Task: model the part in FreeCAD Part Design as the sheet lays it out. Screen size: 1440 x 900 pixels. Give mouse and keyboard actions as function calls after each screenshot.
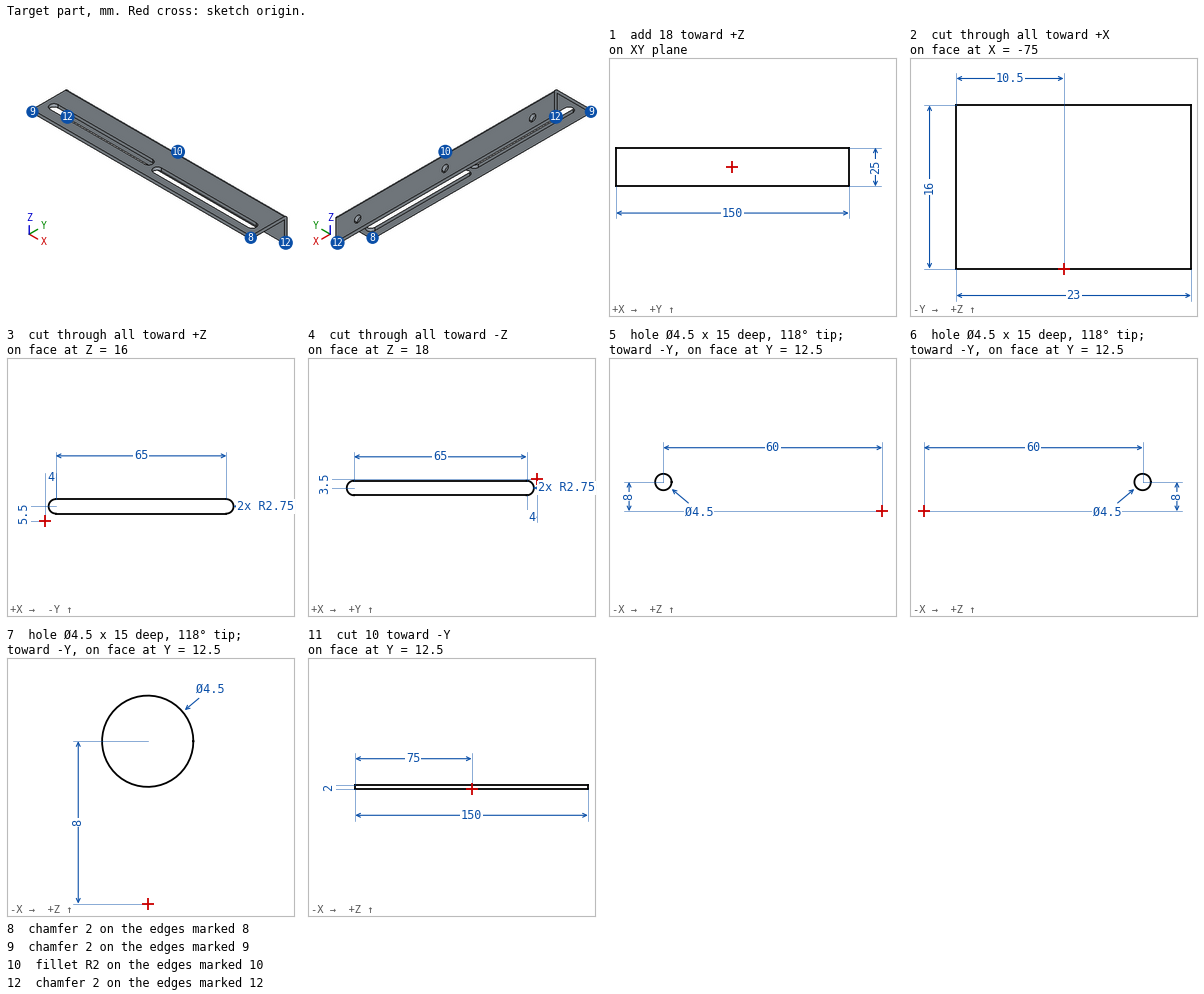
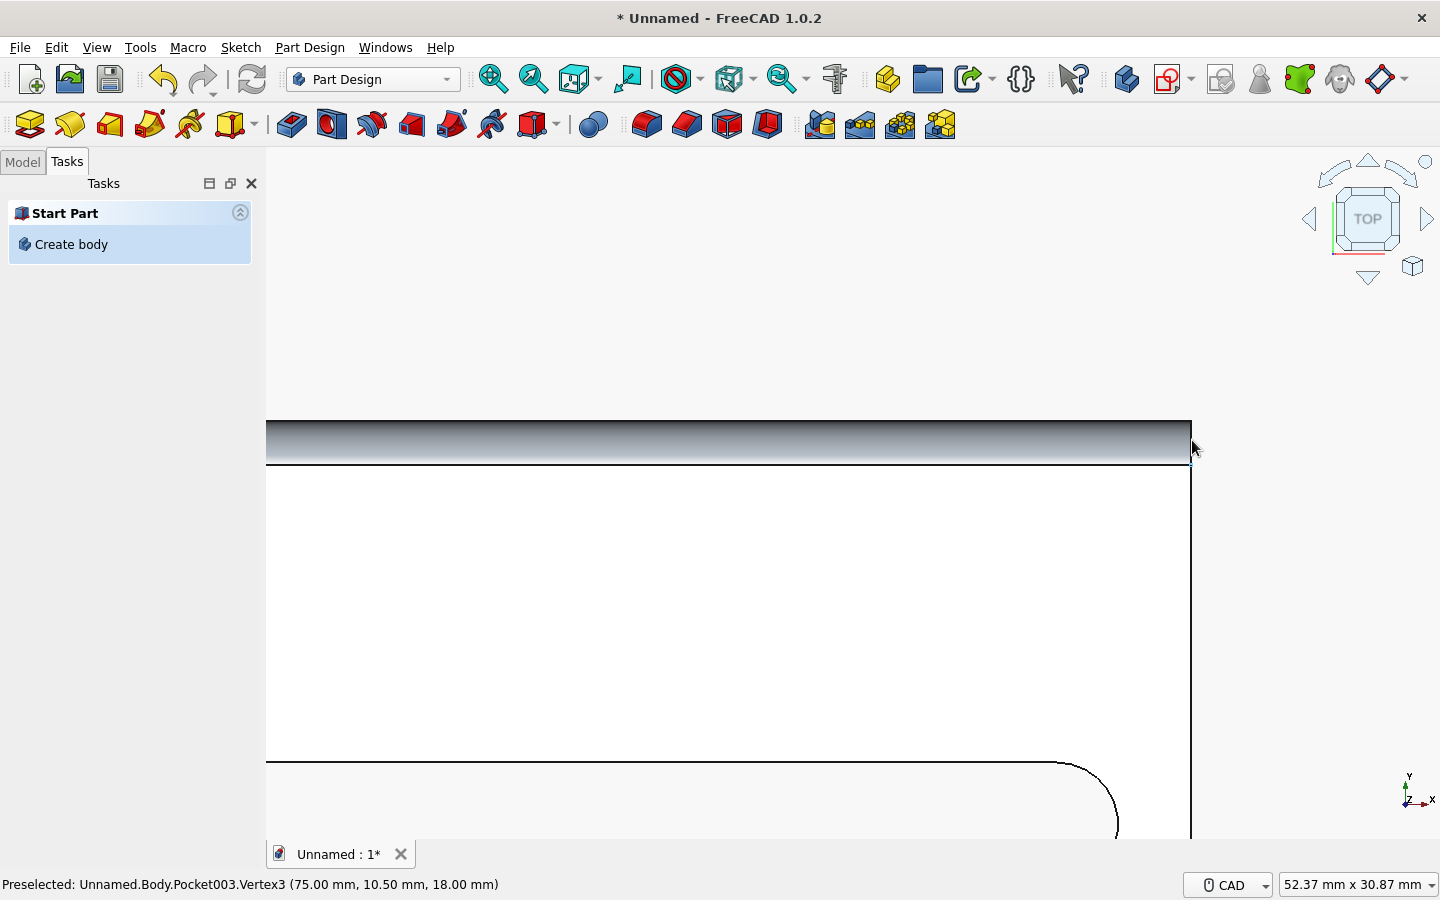
click(494, 80)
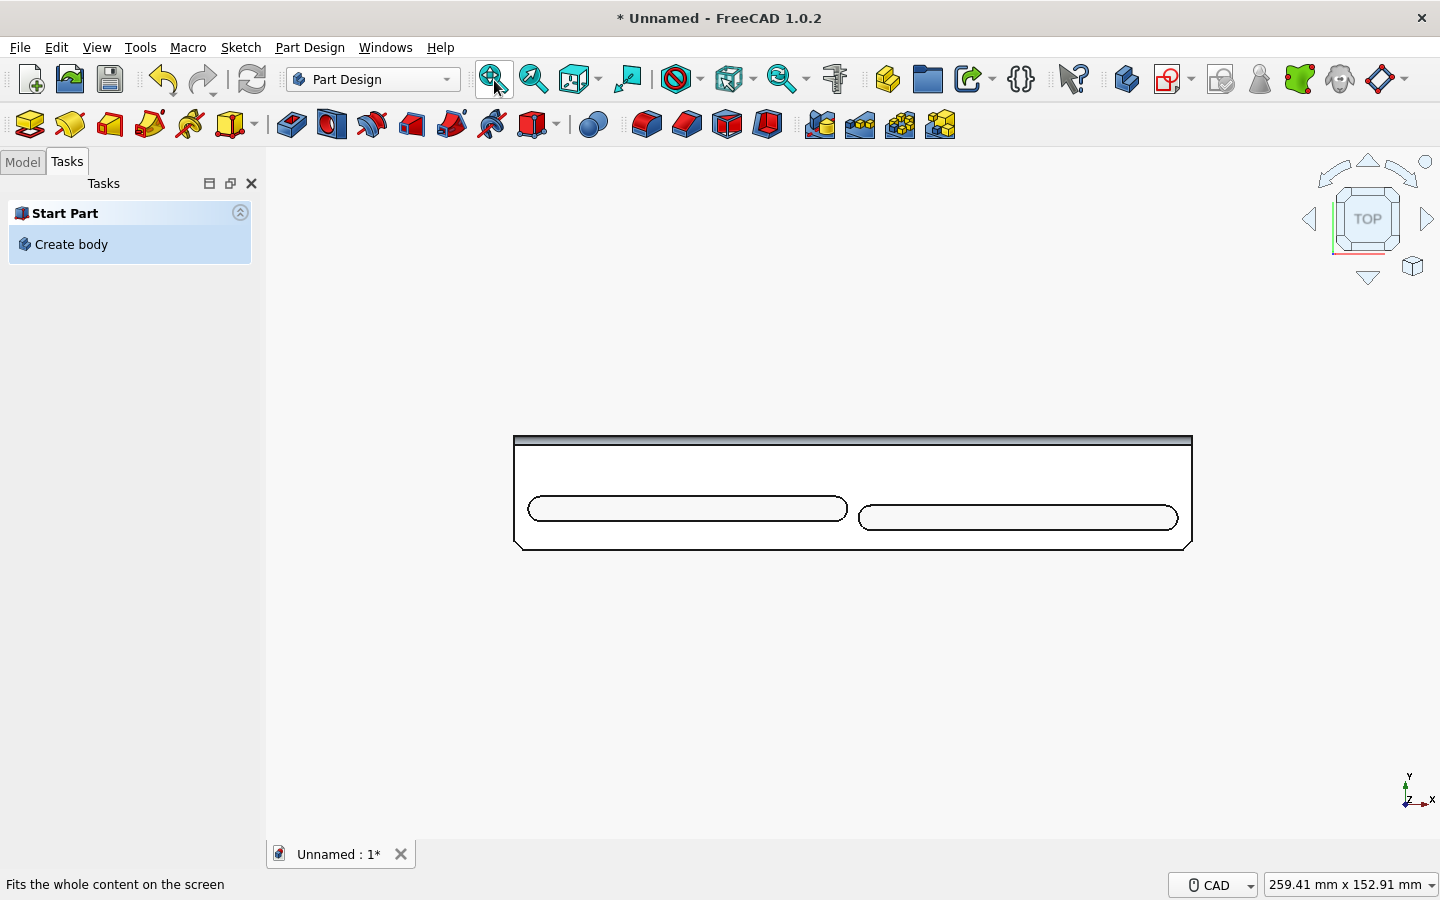
key(1)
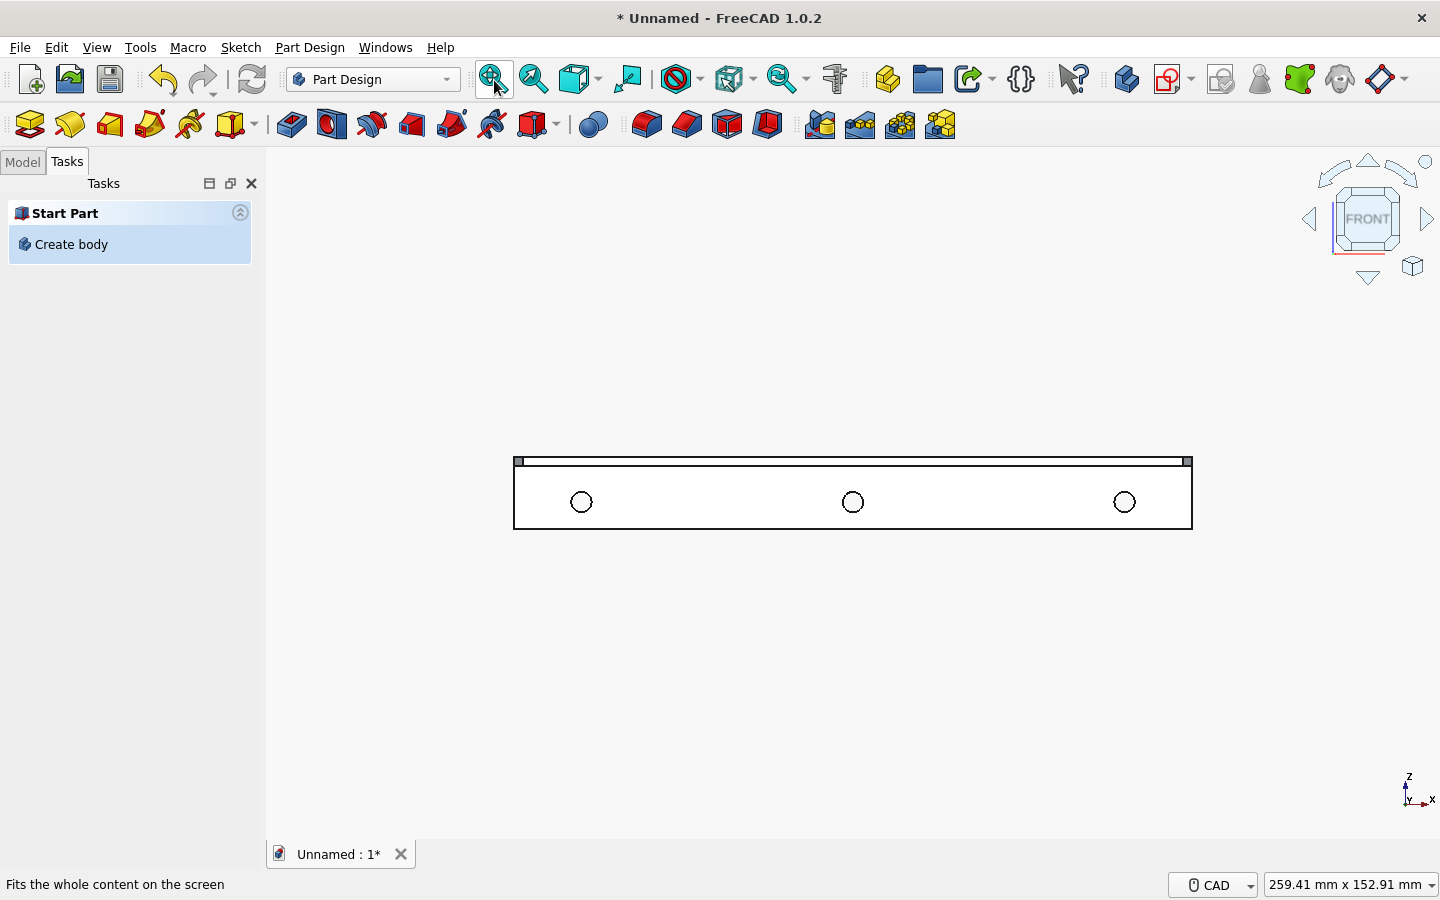
scroll(1192, 528, up, 8)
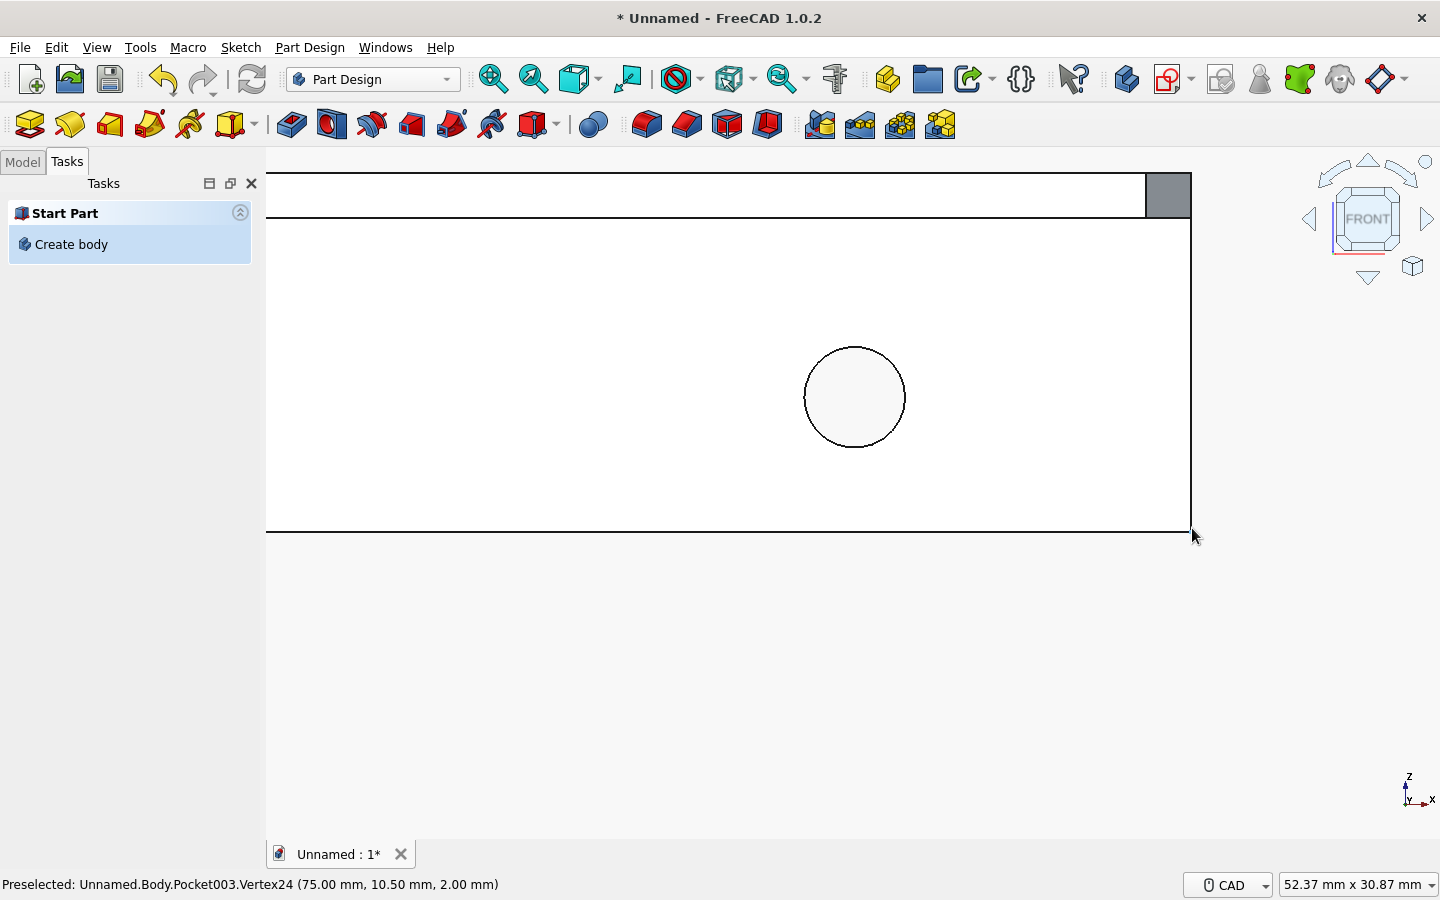
click(494, 80)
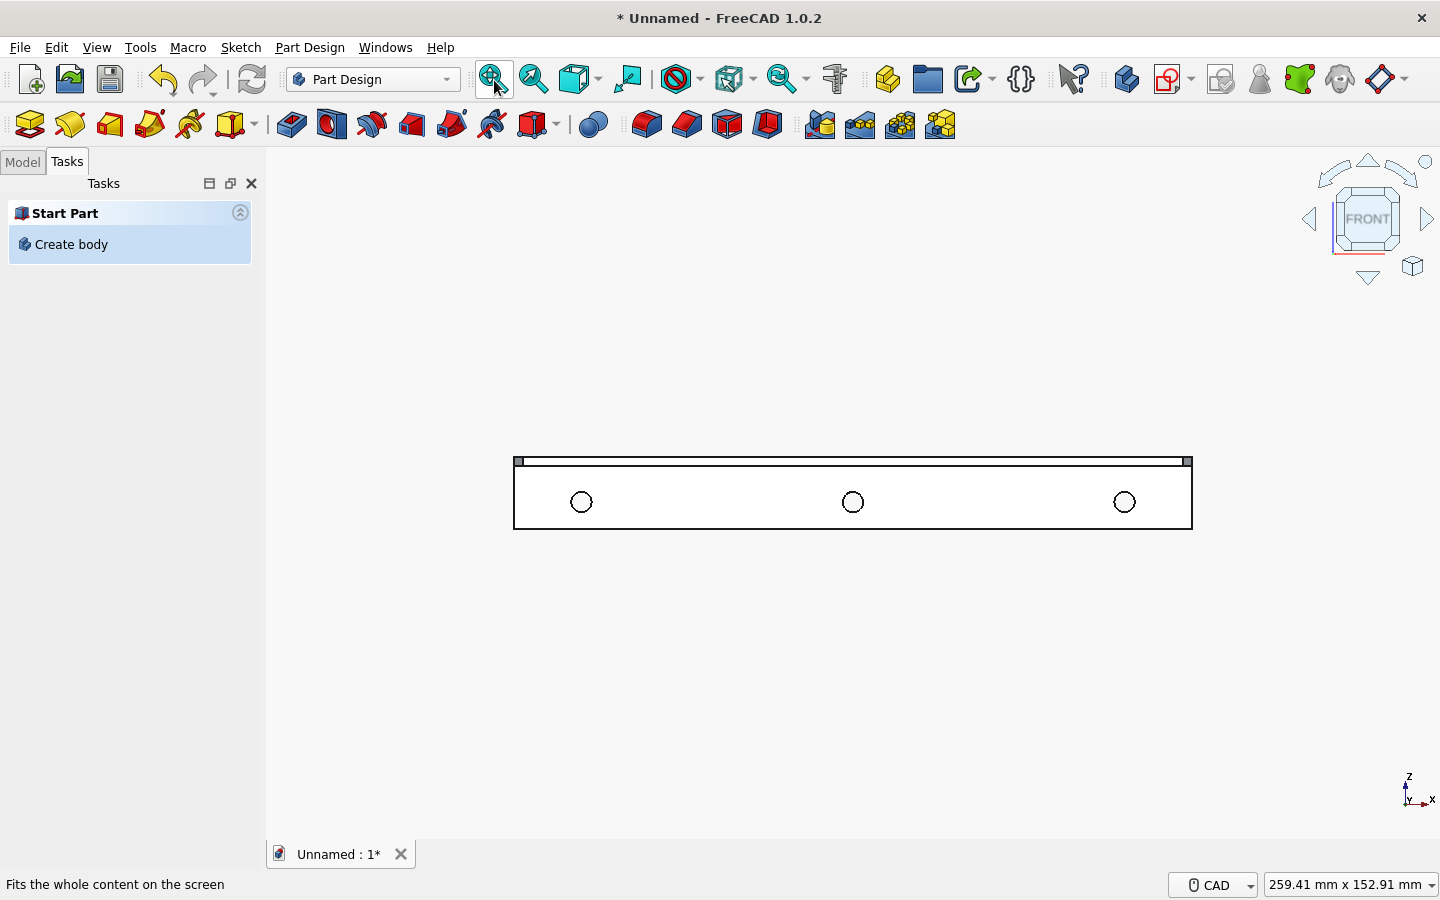
key(3)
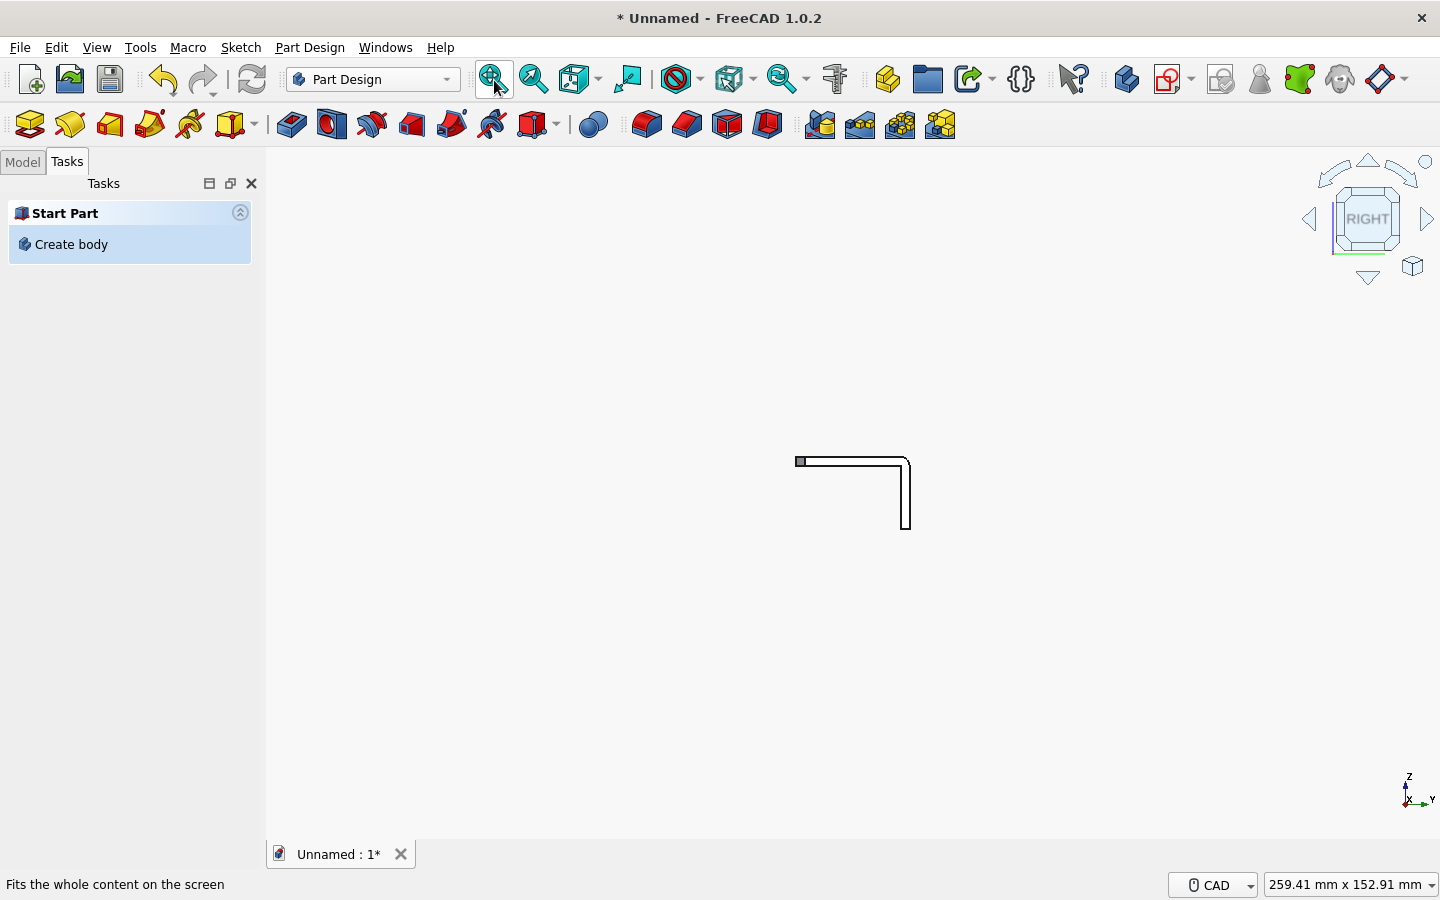
click(494, 80)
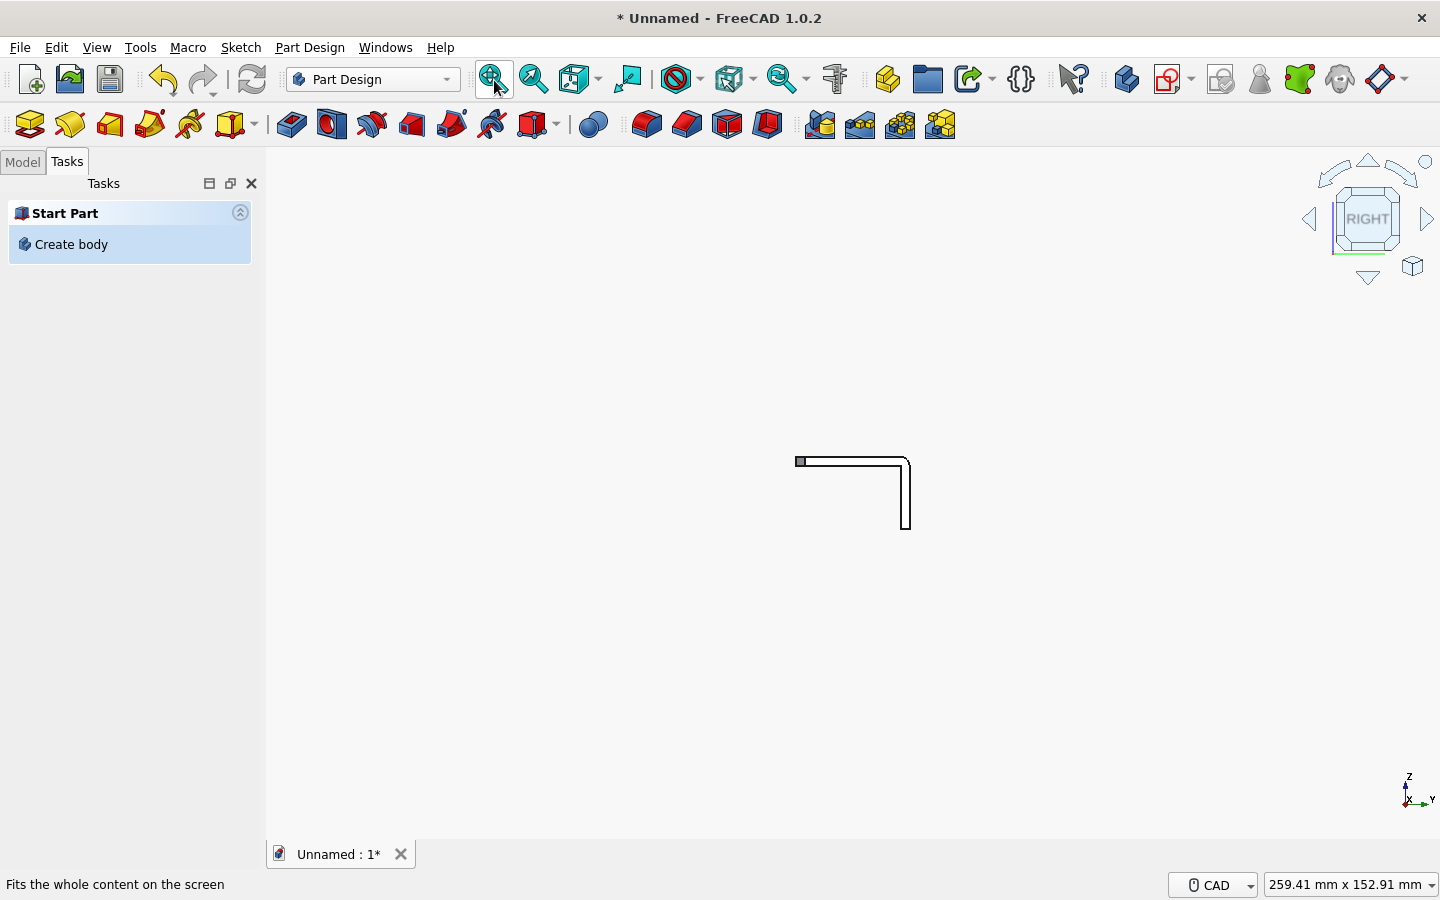
scroll(905, 528, up, 8)